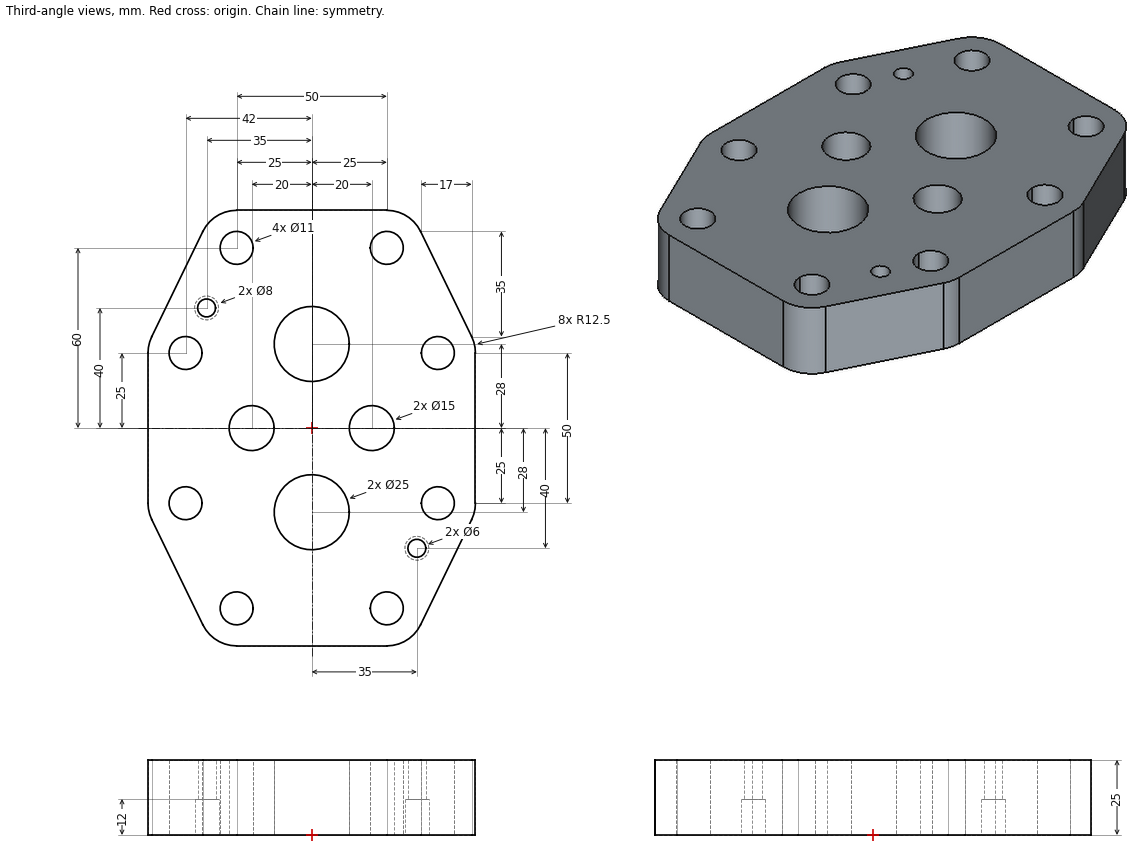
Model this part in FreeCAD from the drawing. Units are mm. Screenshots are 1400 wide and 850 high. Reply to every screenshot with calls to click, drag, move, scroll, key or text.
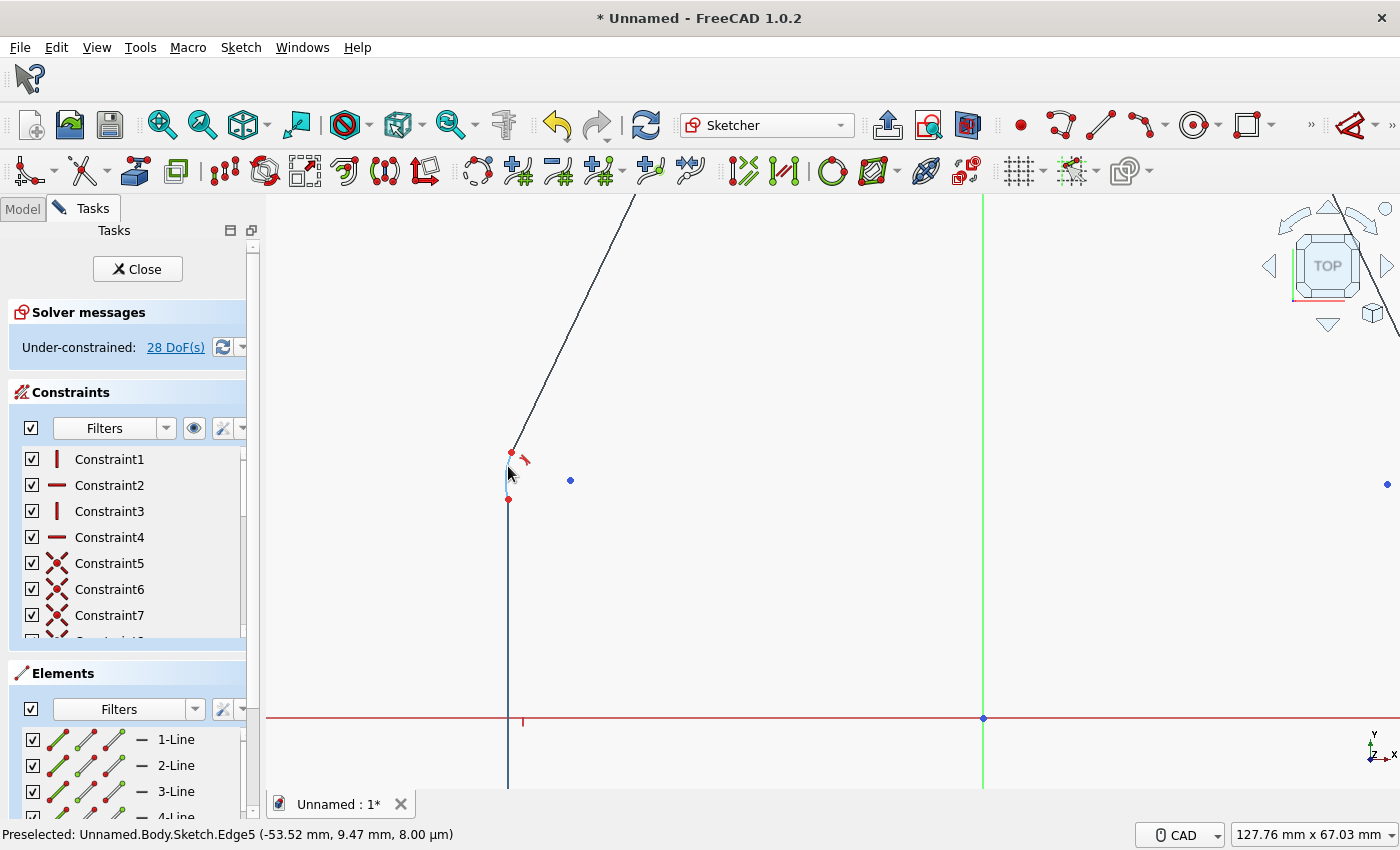
click(507, 466)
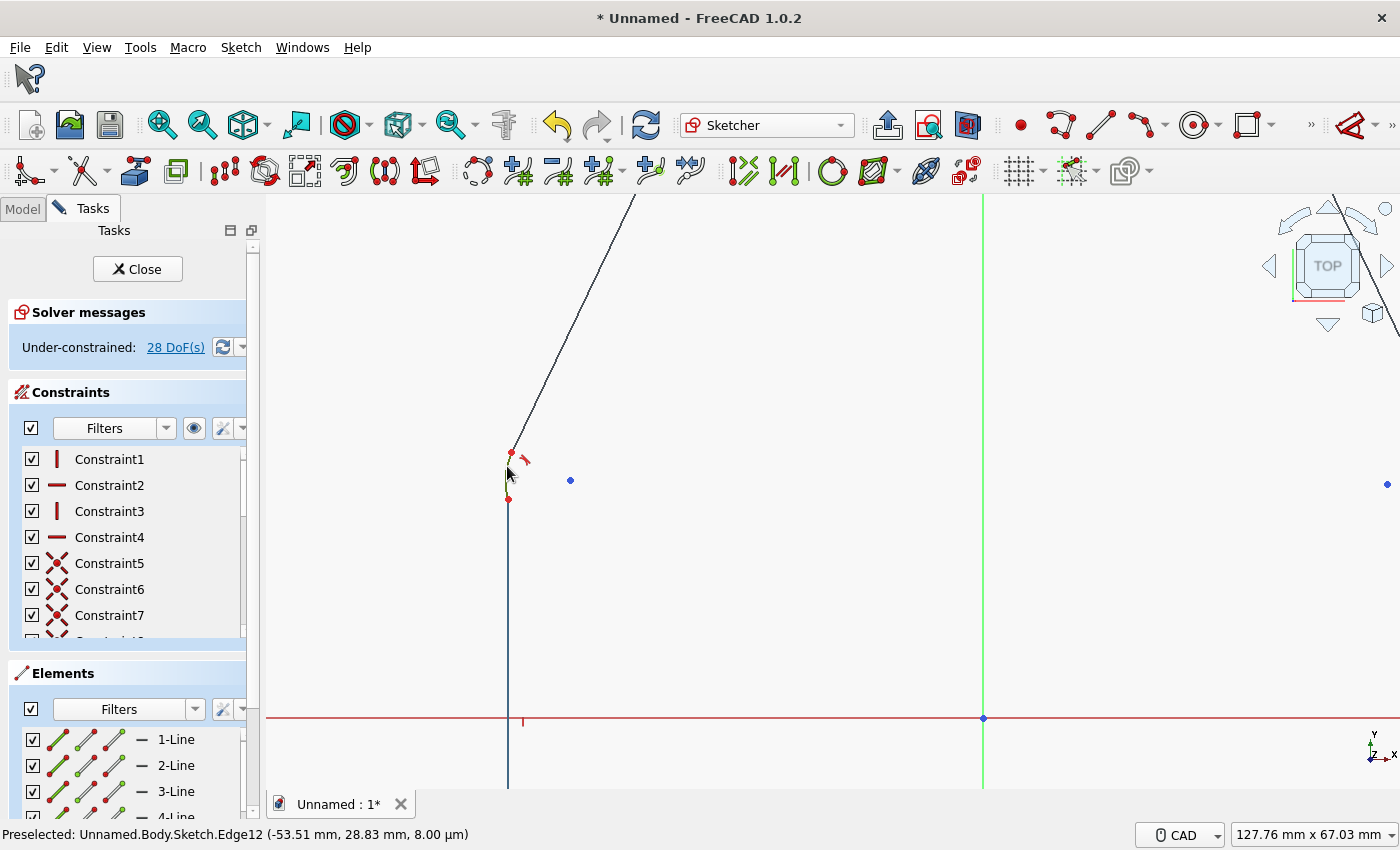
key(t)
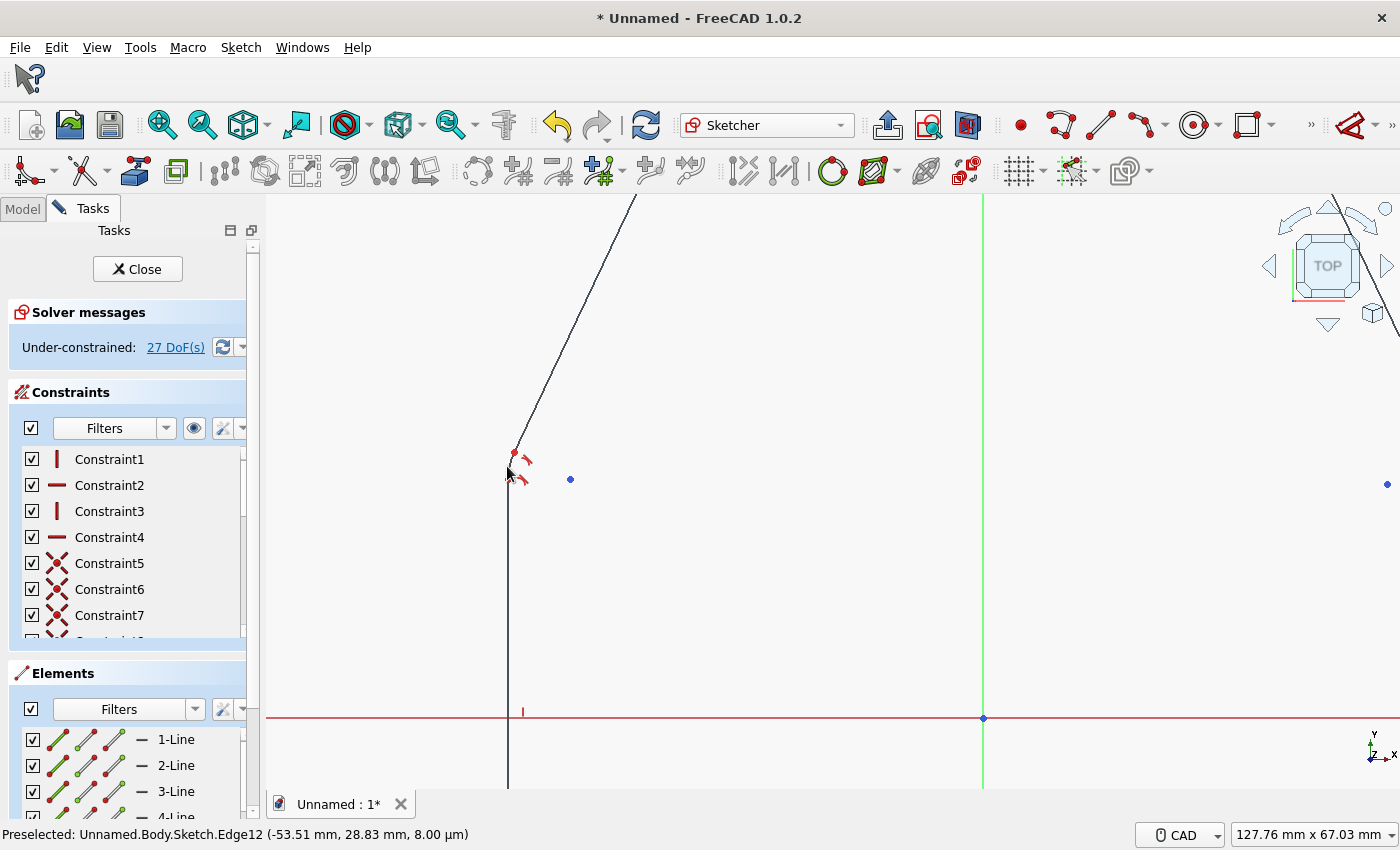
click(508, 619)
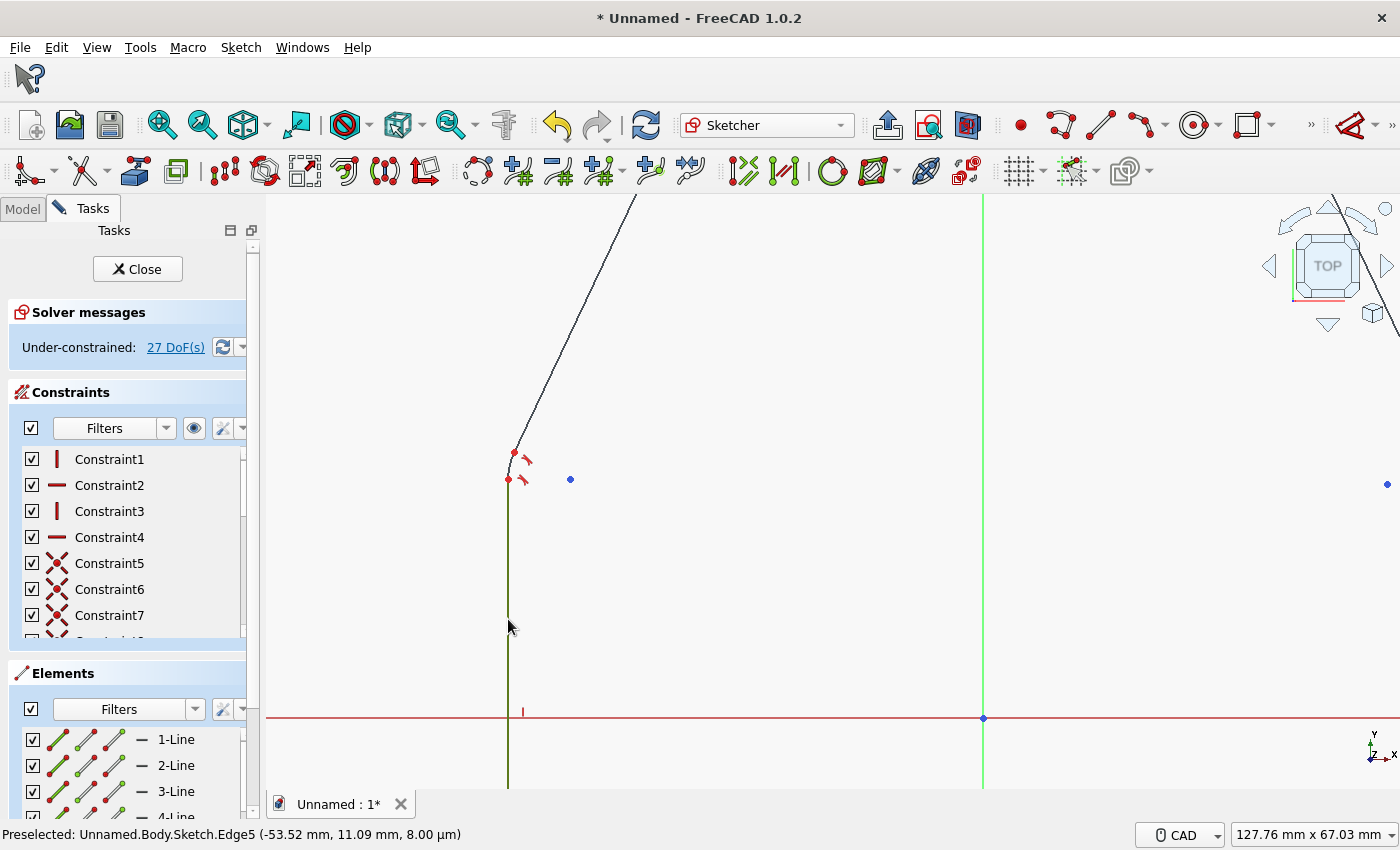
scroll(670, 394, down, 6)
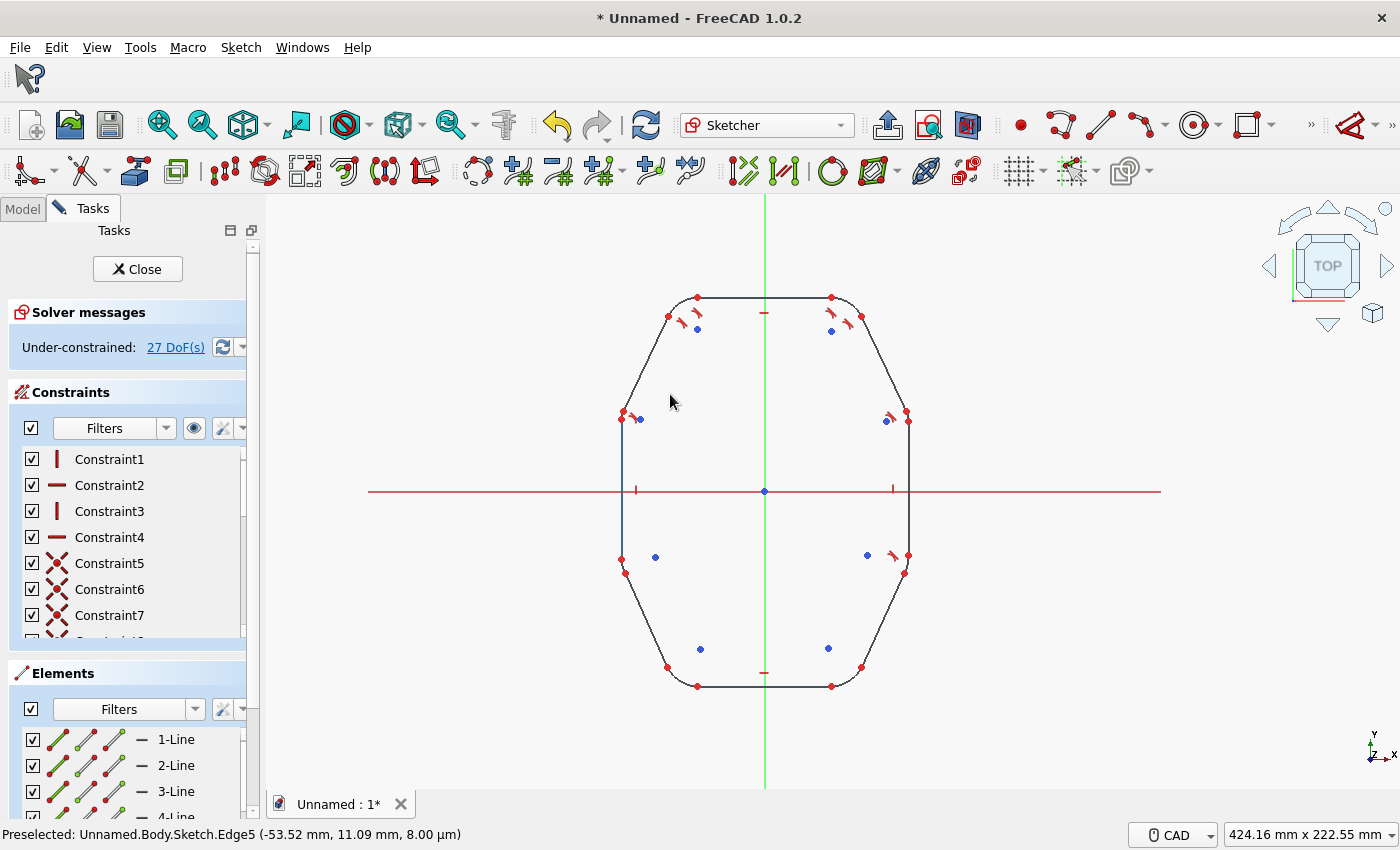
scroll(622, 564, up, 6)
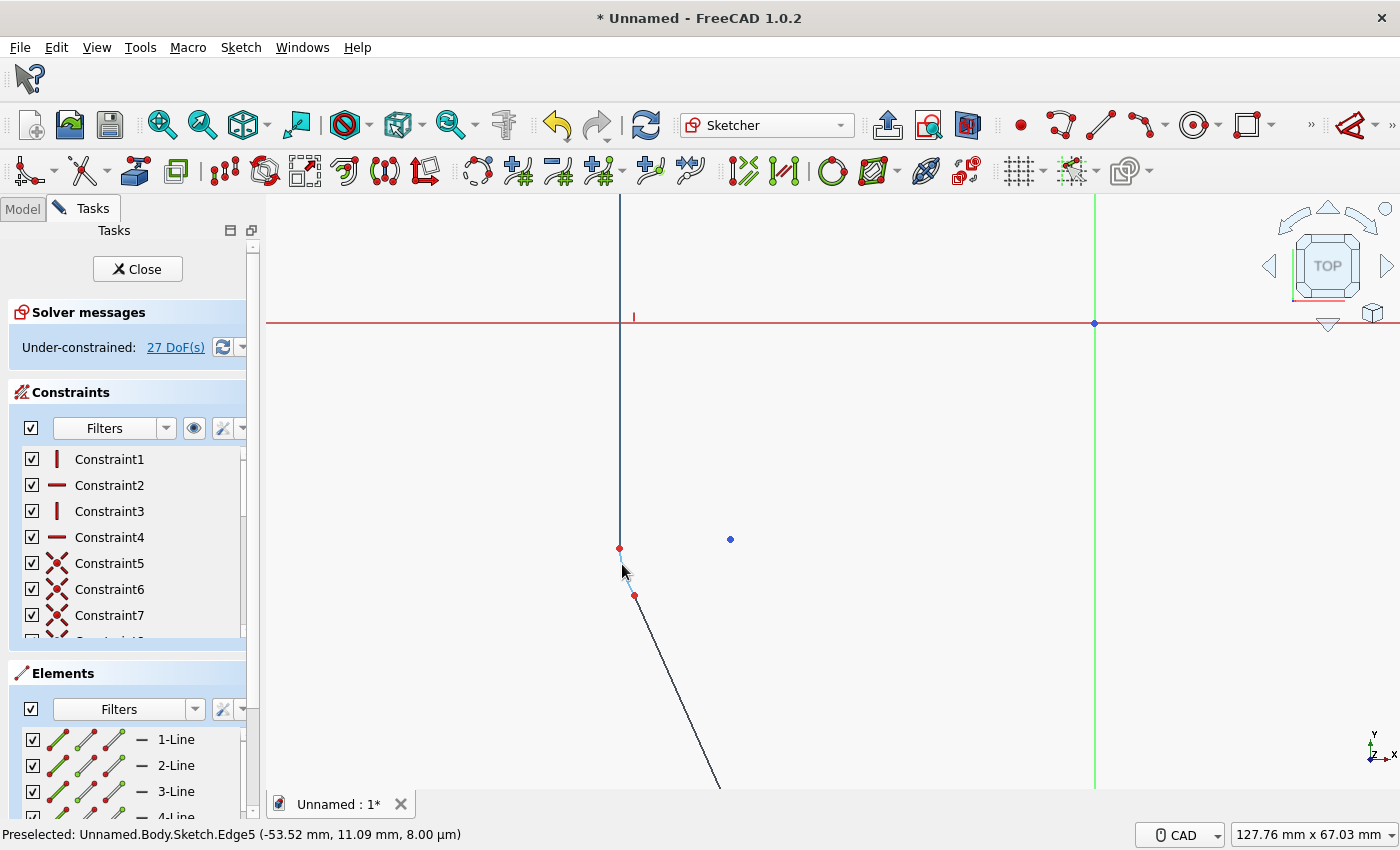
click(622, 563)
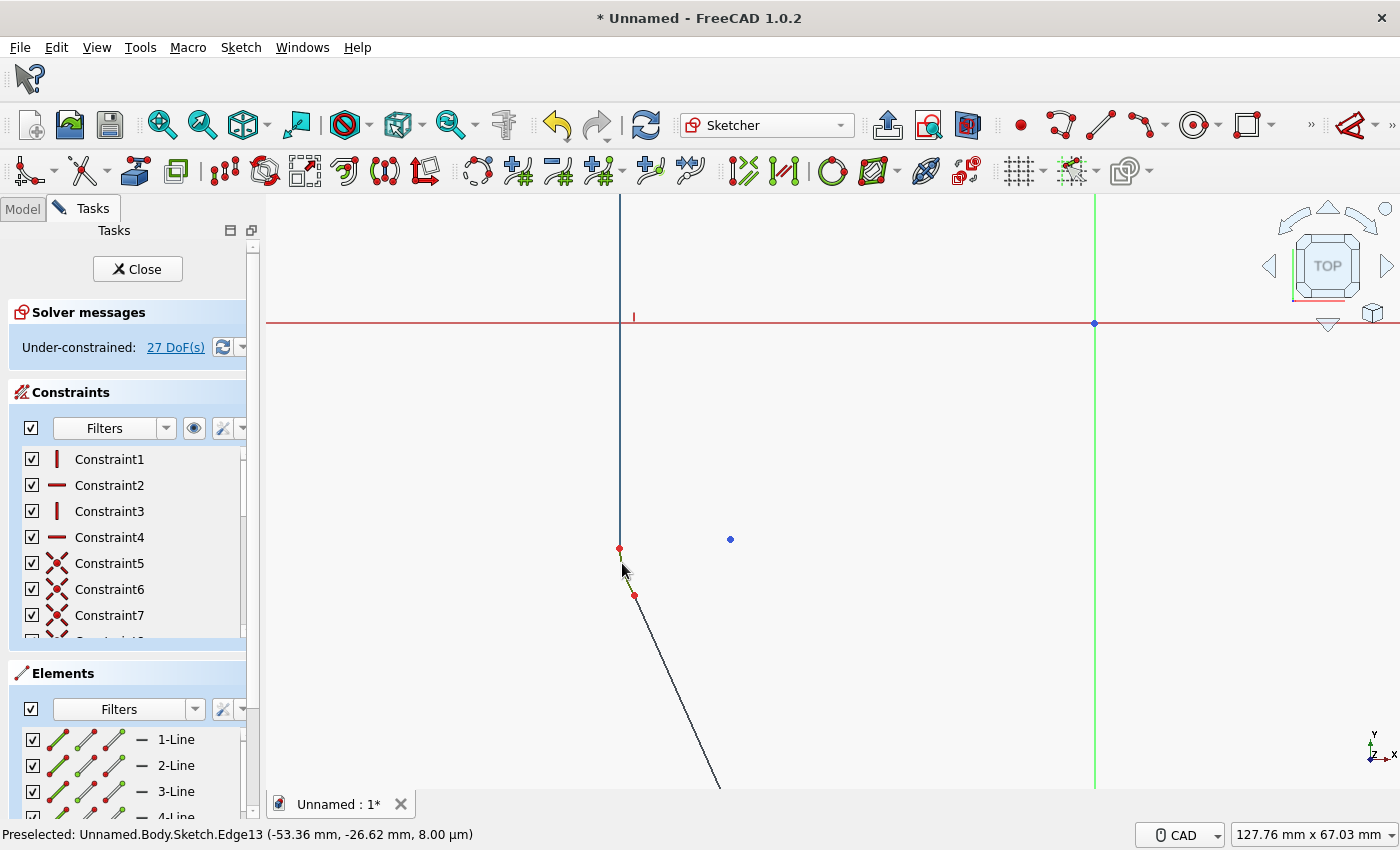
key(t)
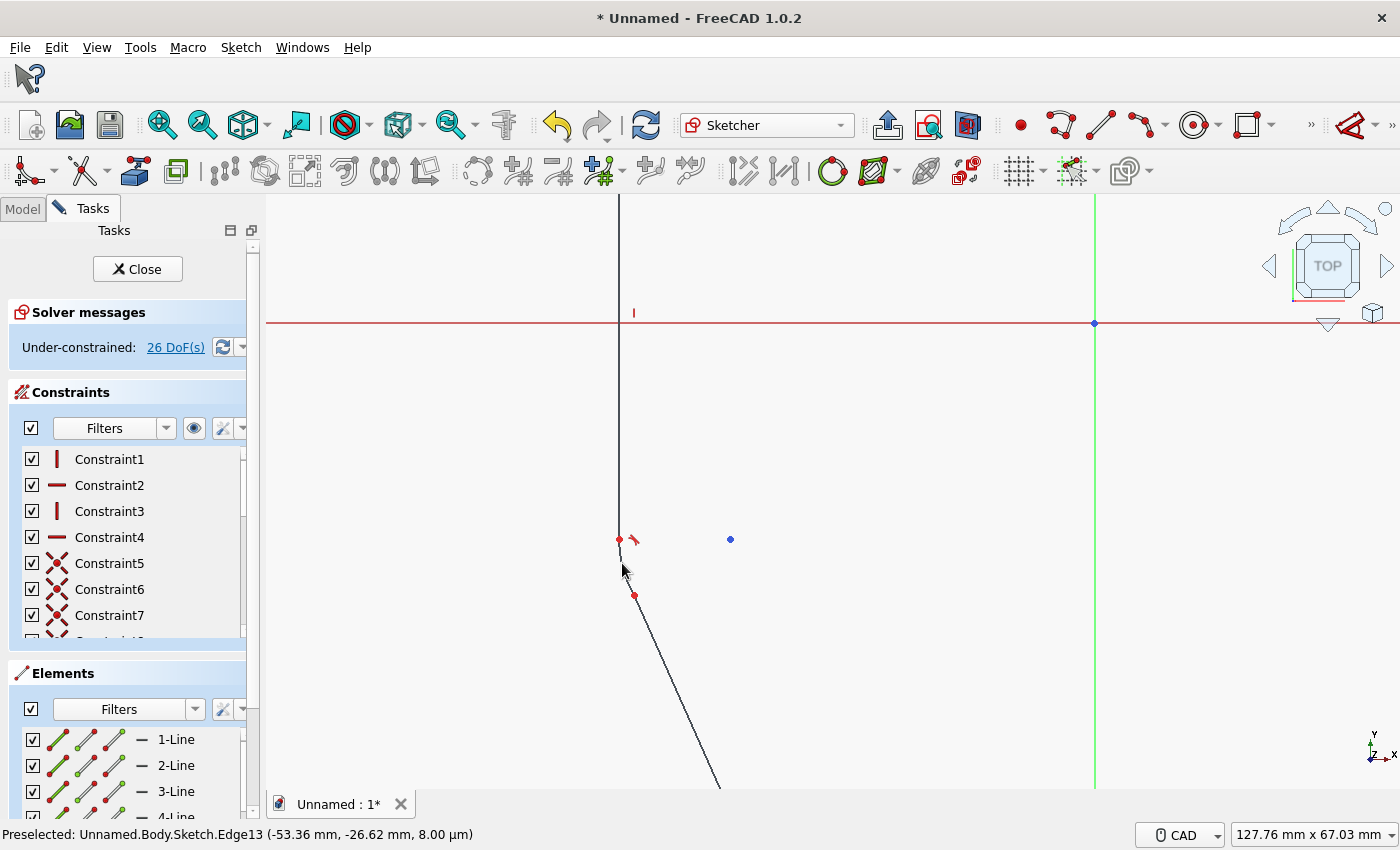
click(676, 689)